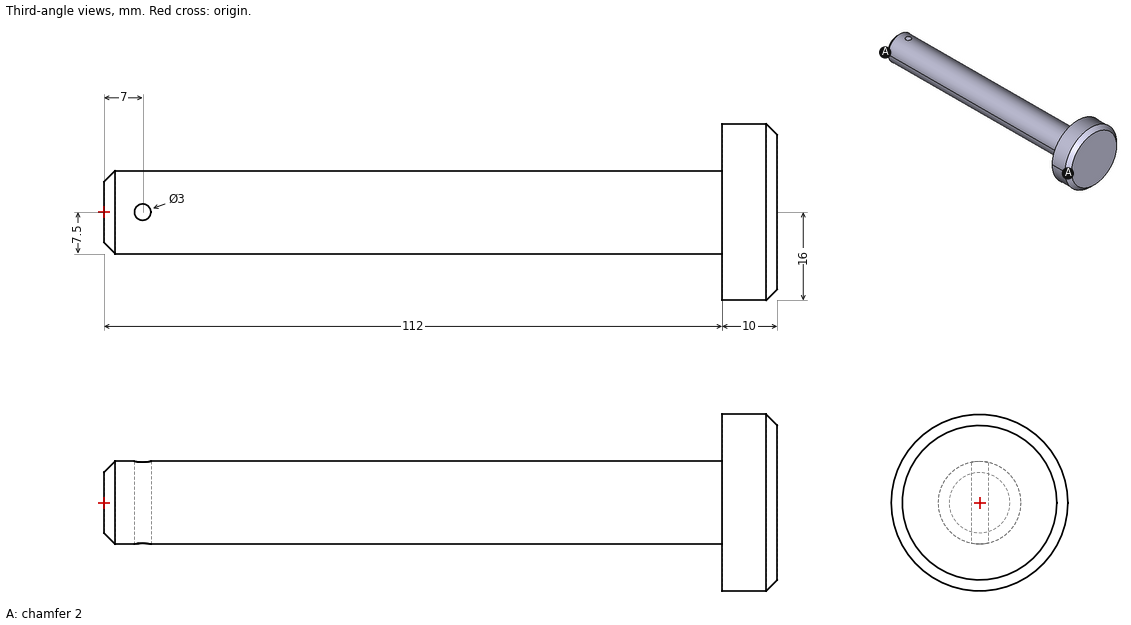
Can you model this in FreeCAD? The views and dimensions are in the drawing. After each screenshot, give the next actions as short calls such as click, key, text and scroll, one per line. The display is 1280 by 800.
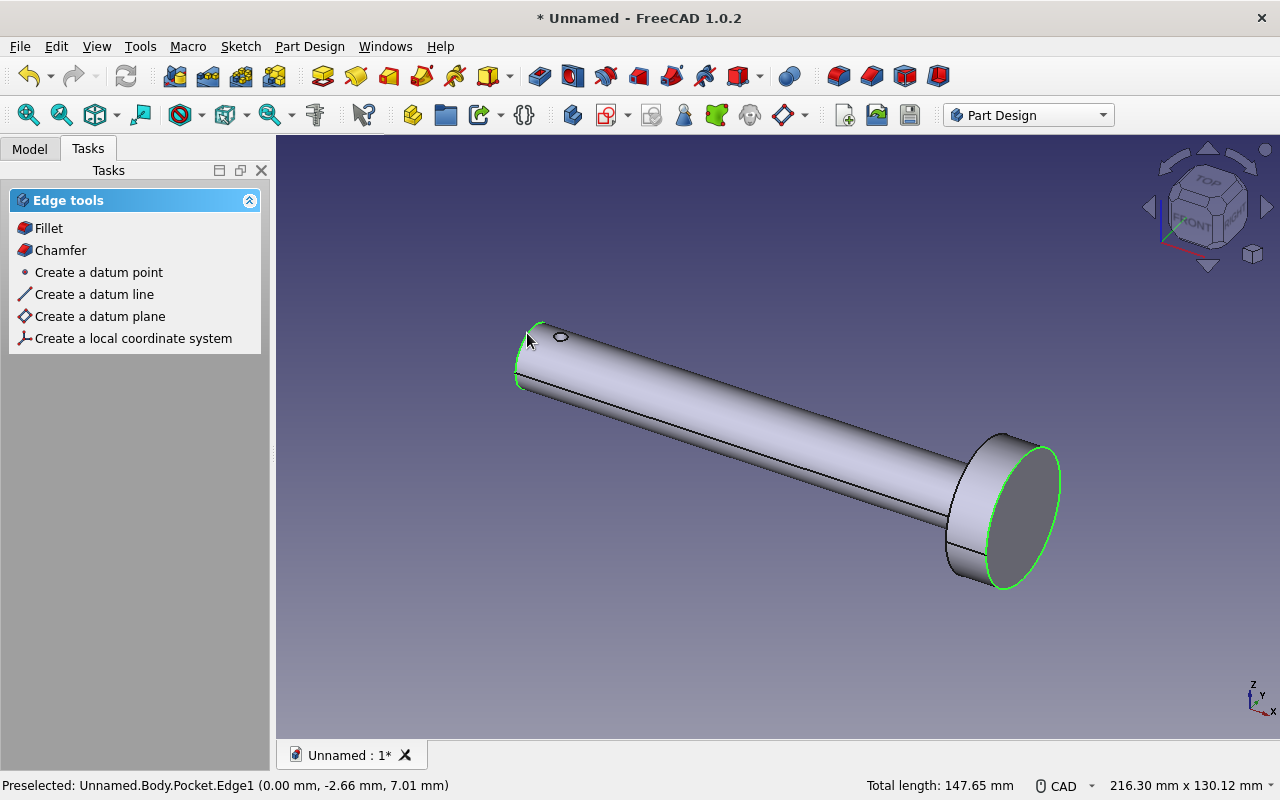
click(872, 76)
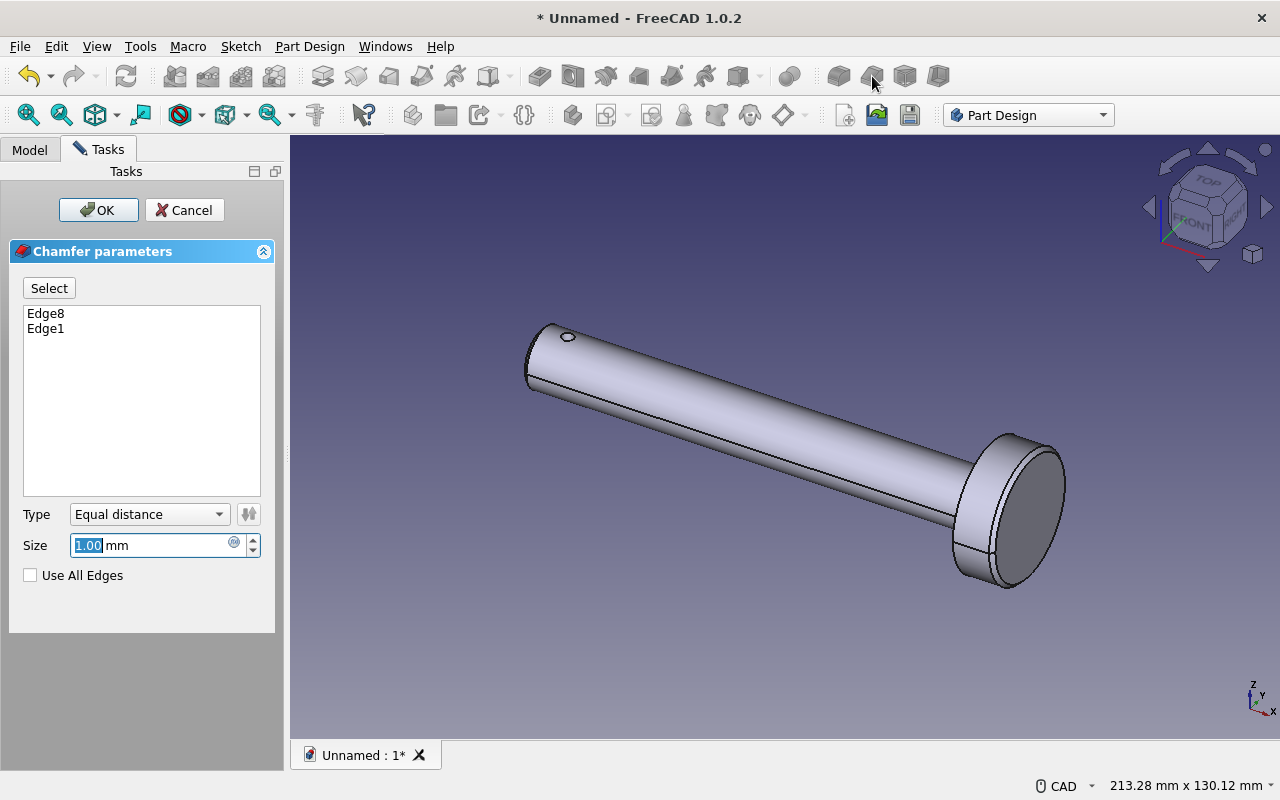
text(2)
key(Tab)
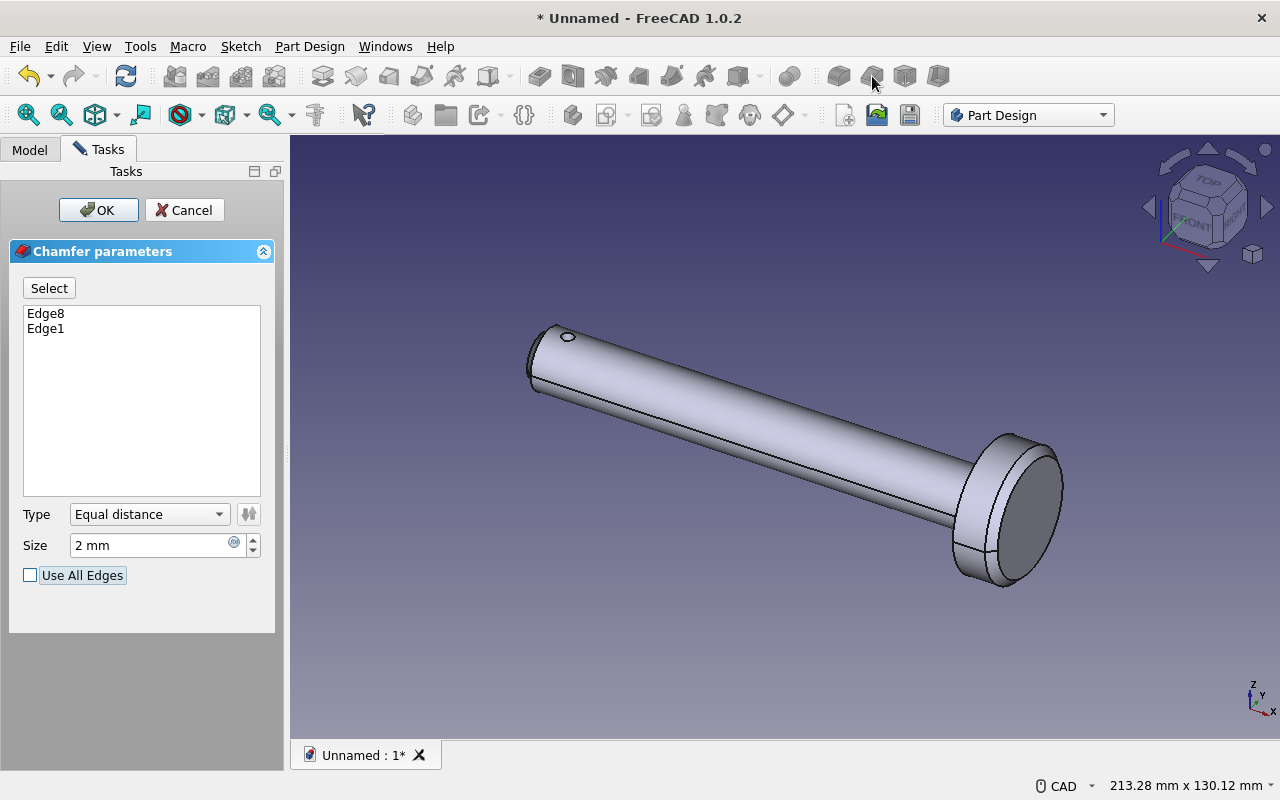
click(99, 210)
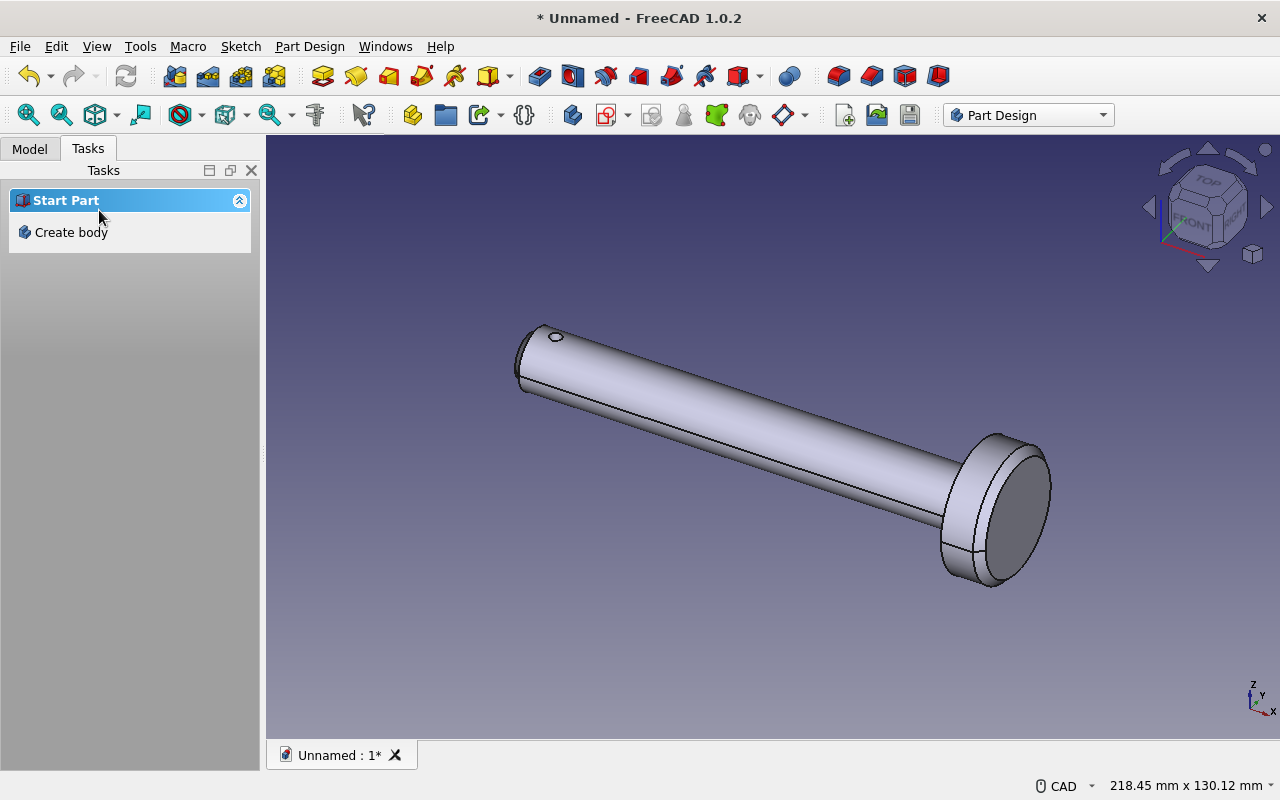
key(0)